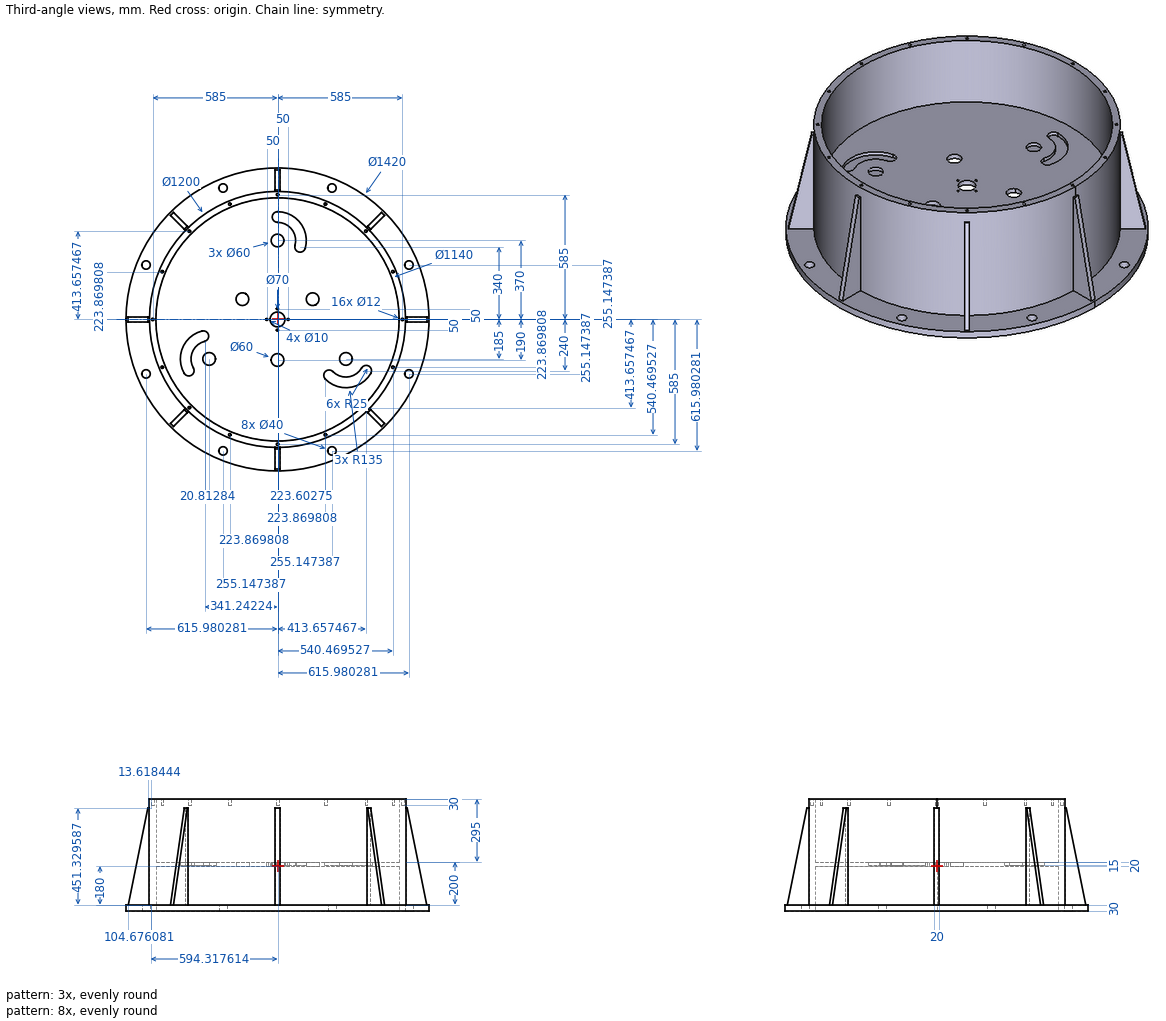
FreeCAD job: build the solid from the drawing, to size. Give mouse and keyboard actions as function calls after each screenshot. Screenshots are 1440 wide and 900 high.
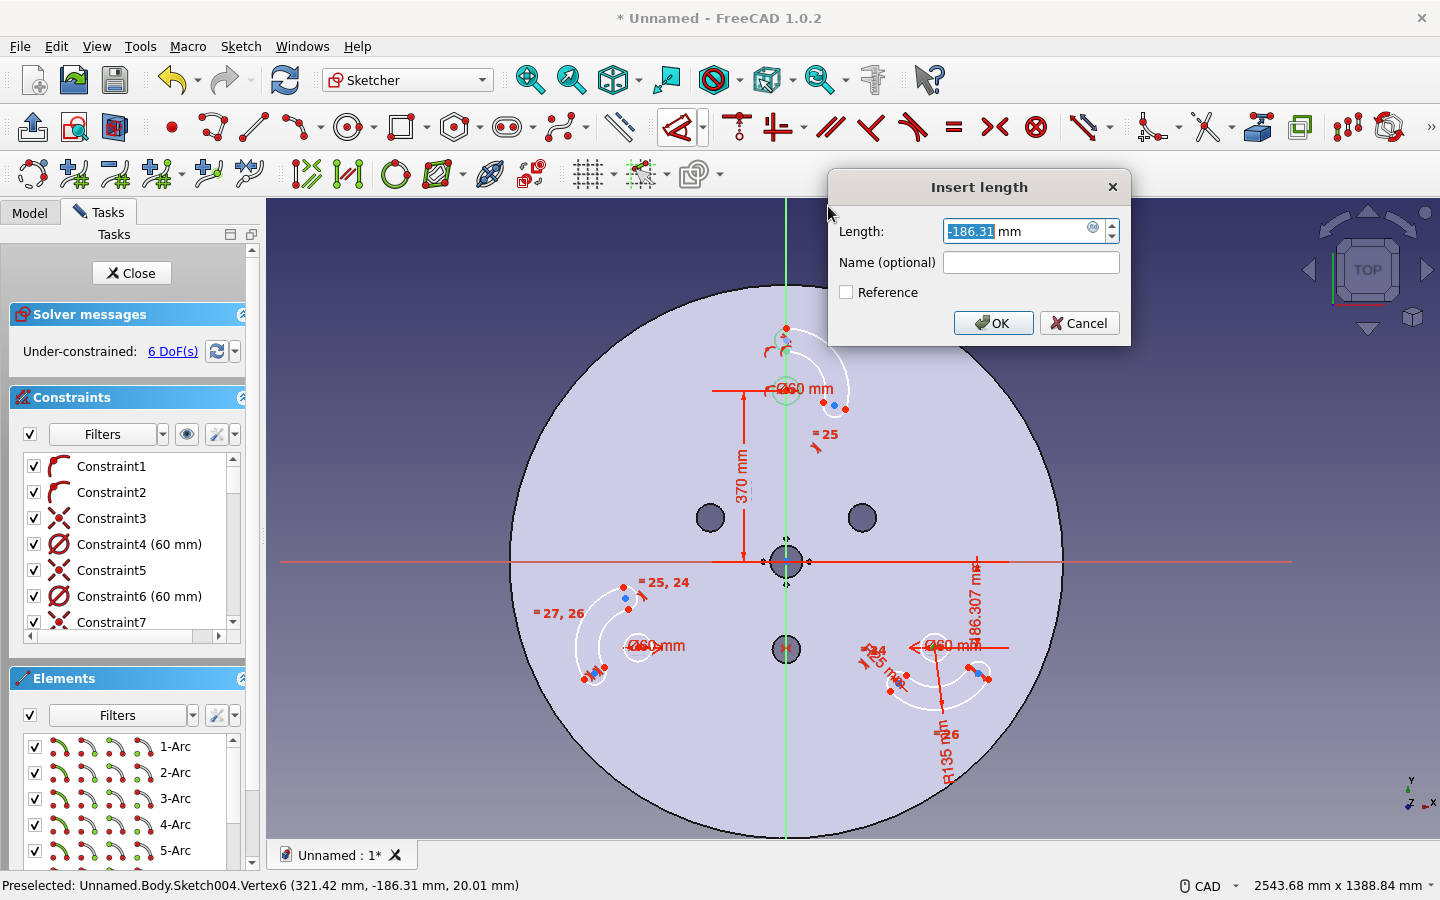
text(-185)
key(Return)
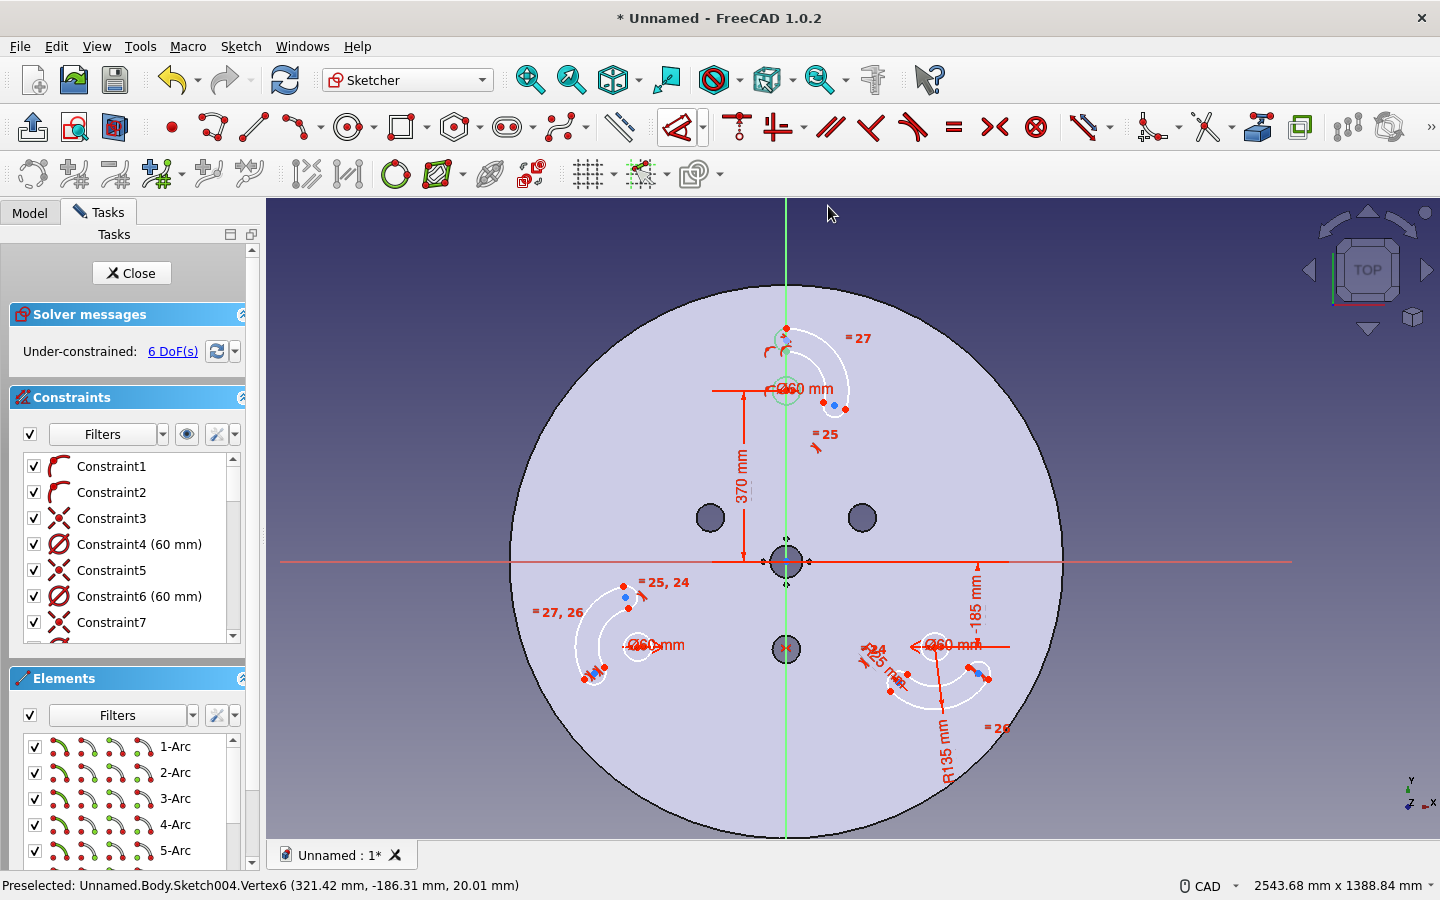
click(979, 673)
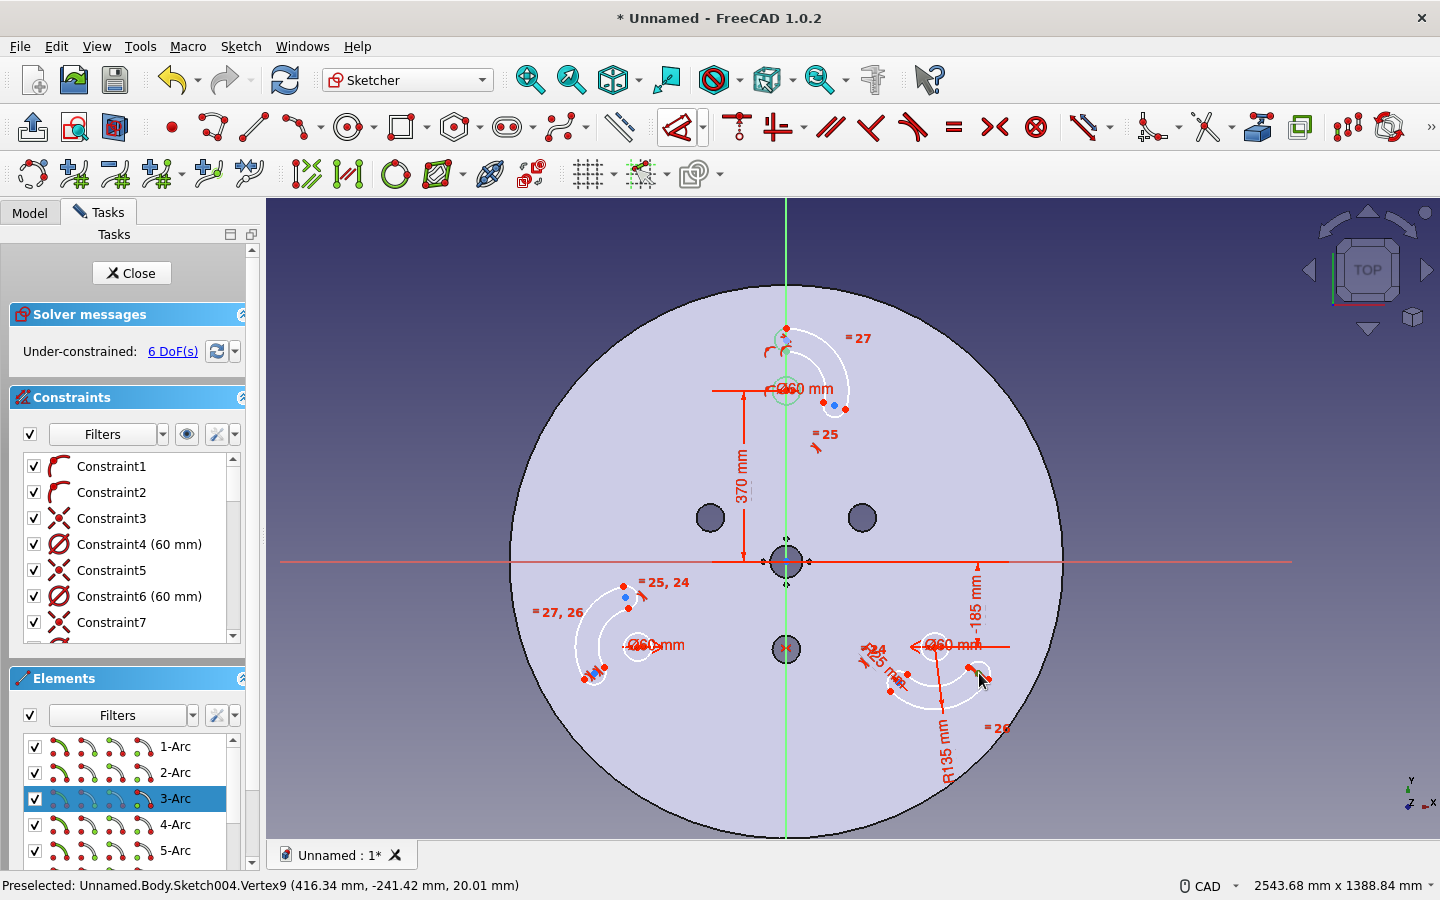
key(i)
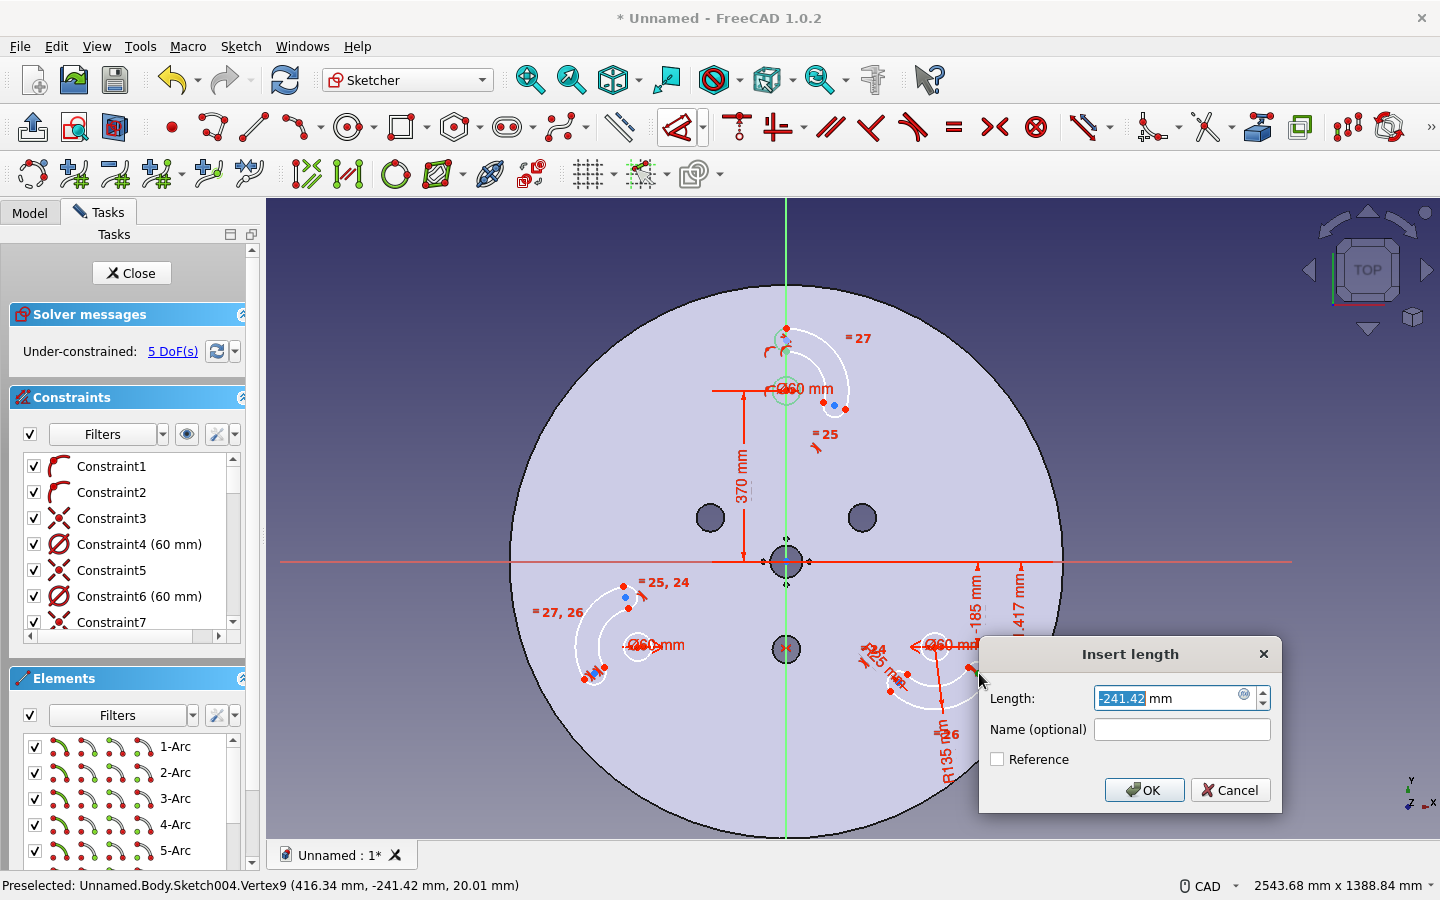
text(-240)
key(Return)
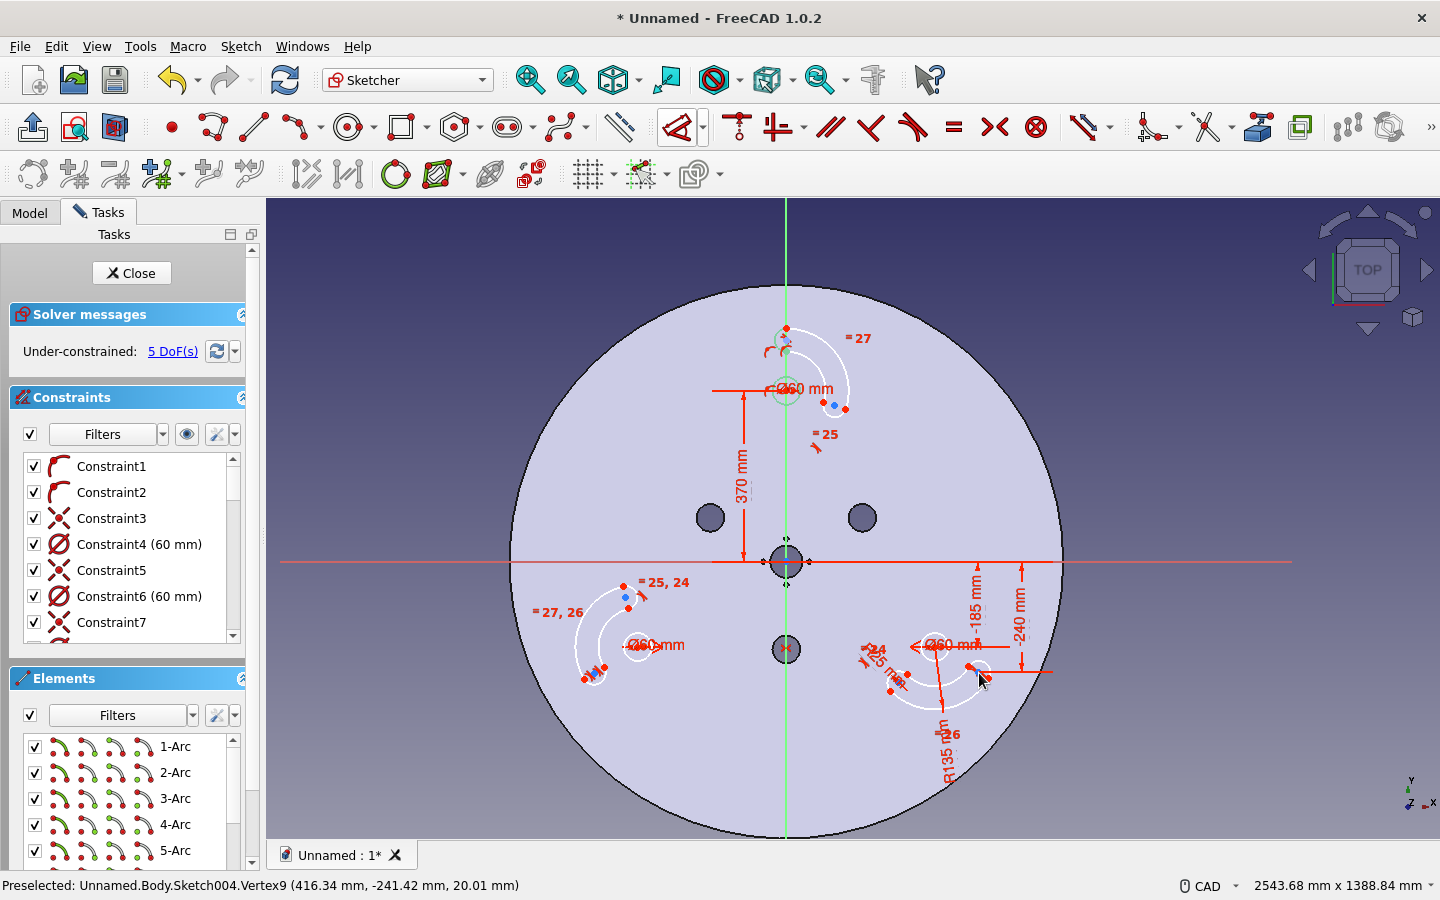
click(594, 673)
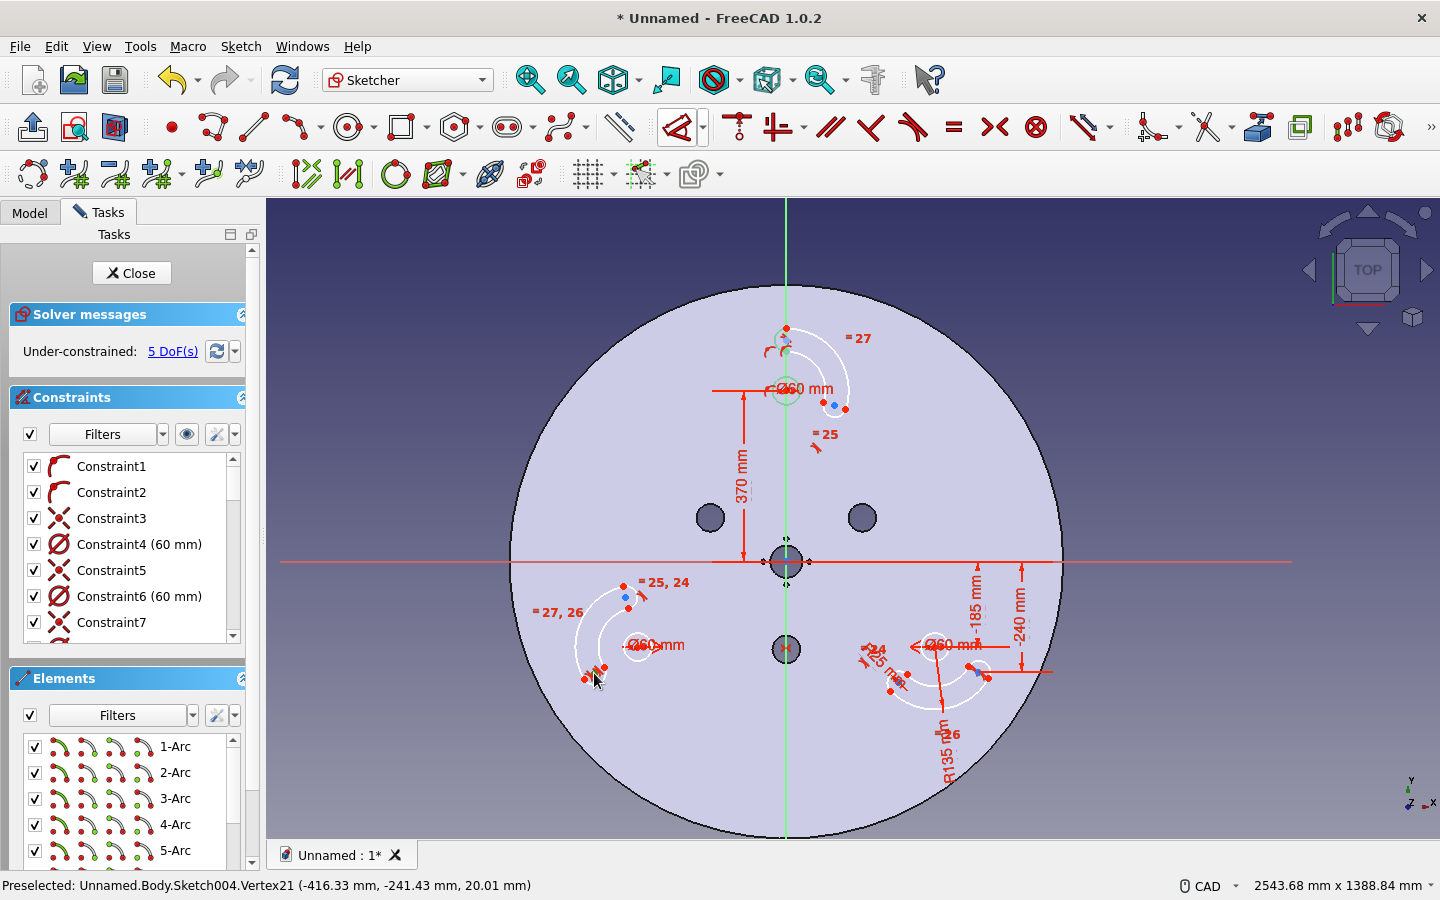
key(i)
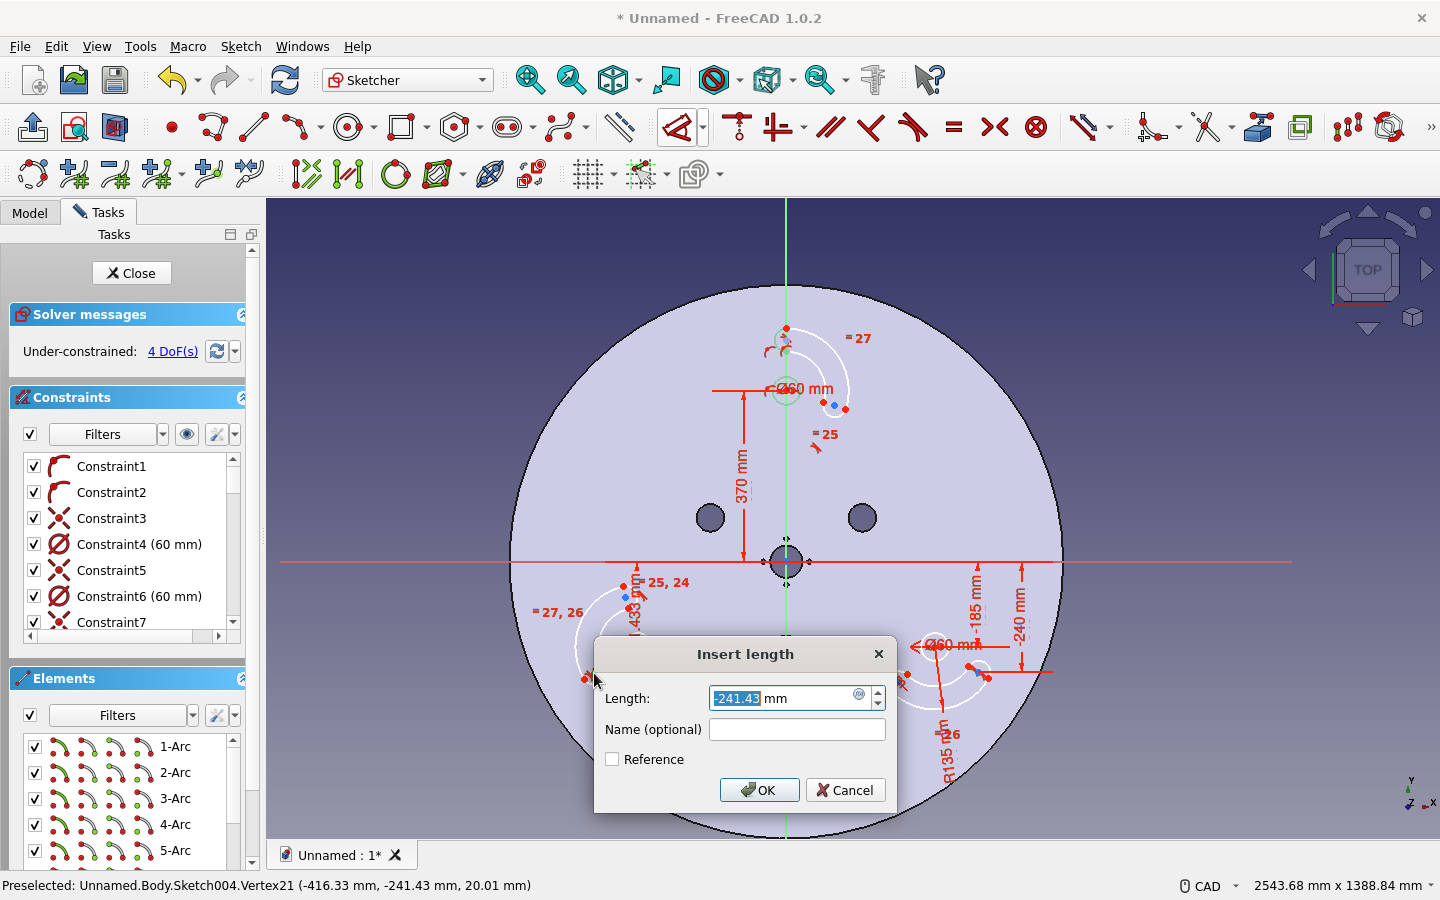
text(-240)
key(Return)